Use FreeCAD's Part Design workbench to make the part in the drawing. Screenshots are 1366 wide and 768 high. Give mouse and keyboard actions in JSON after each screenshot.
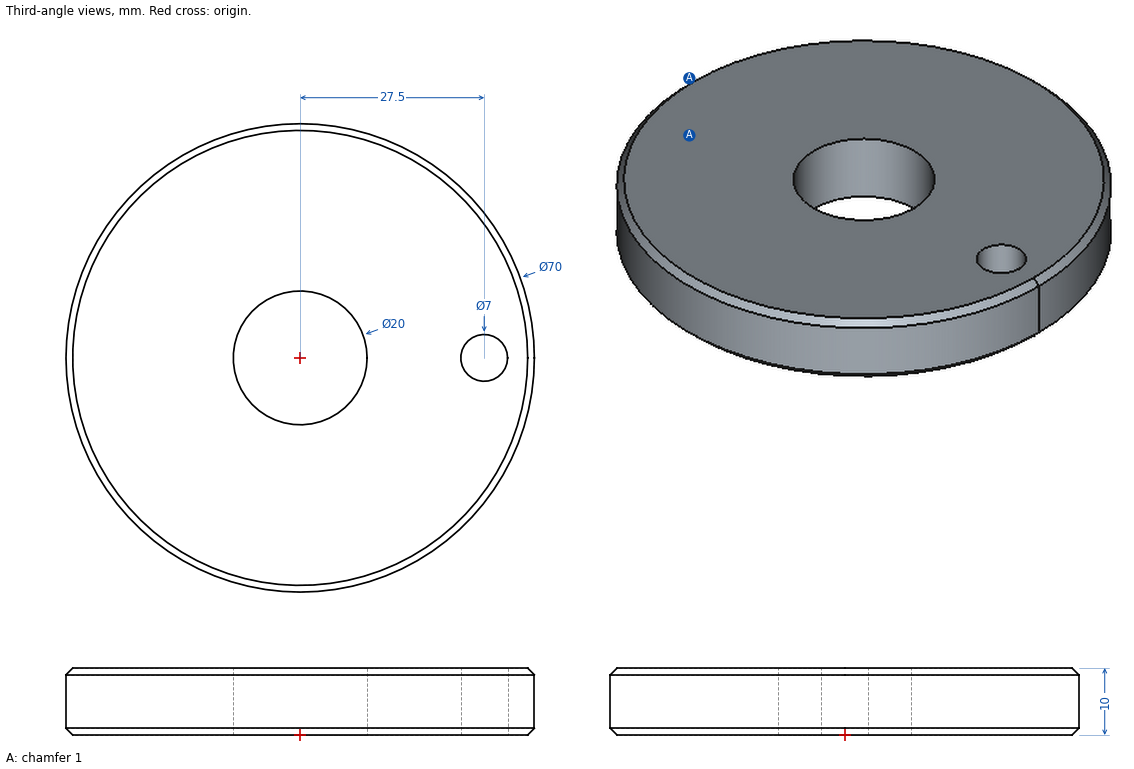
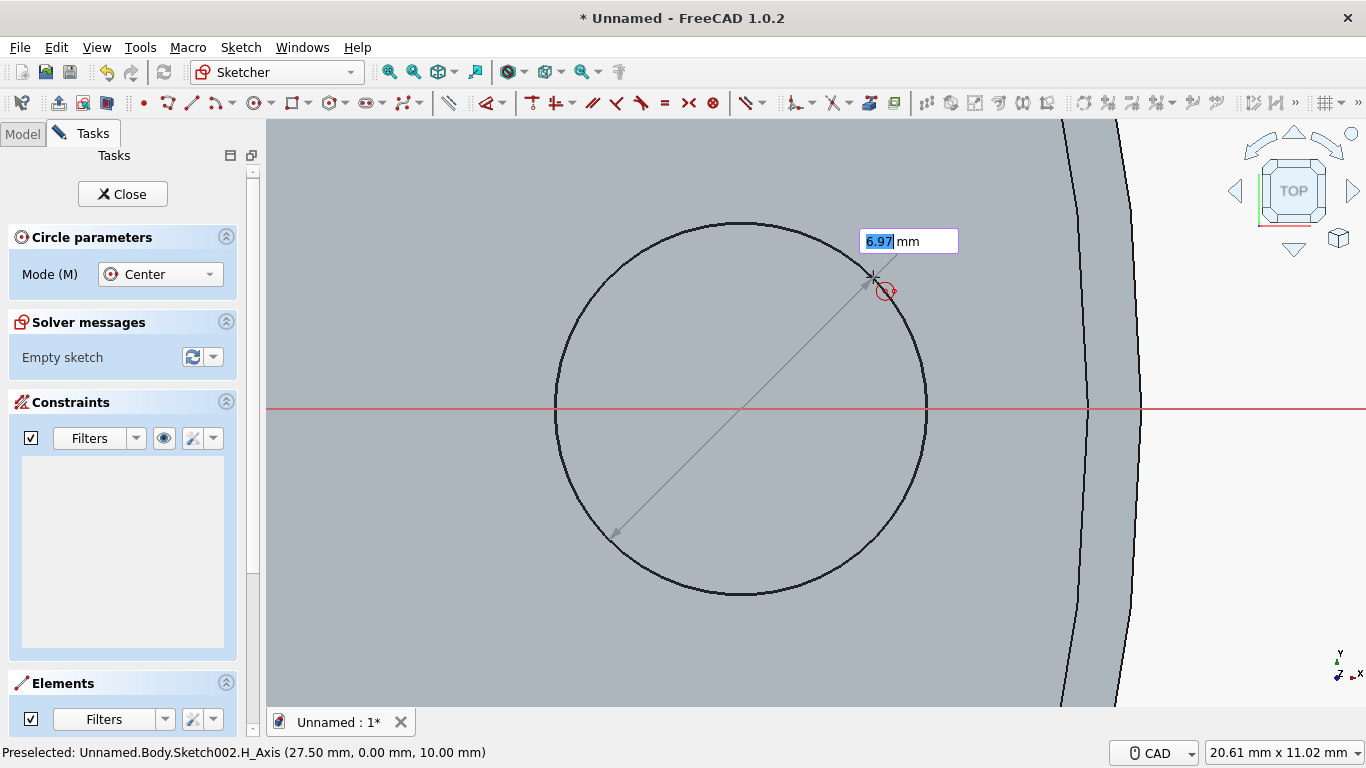
{"action": "type", "text": "7"}
{"action": "key", "text": "Return"}
{"action": "key", "text": "Escape"}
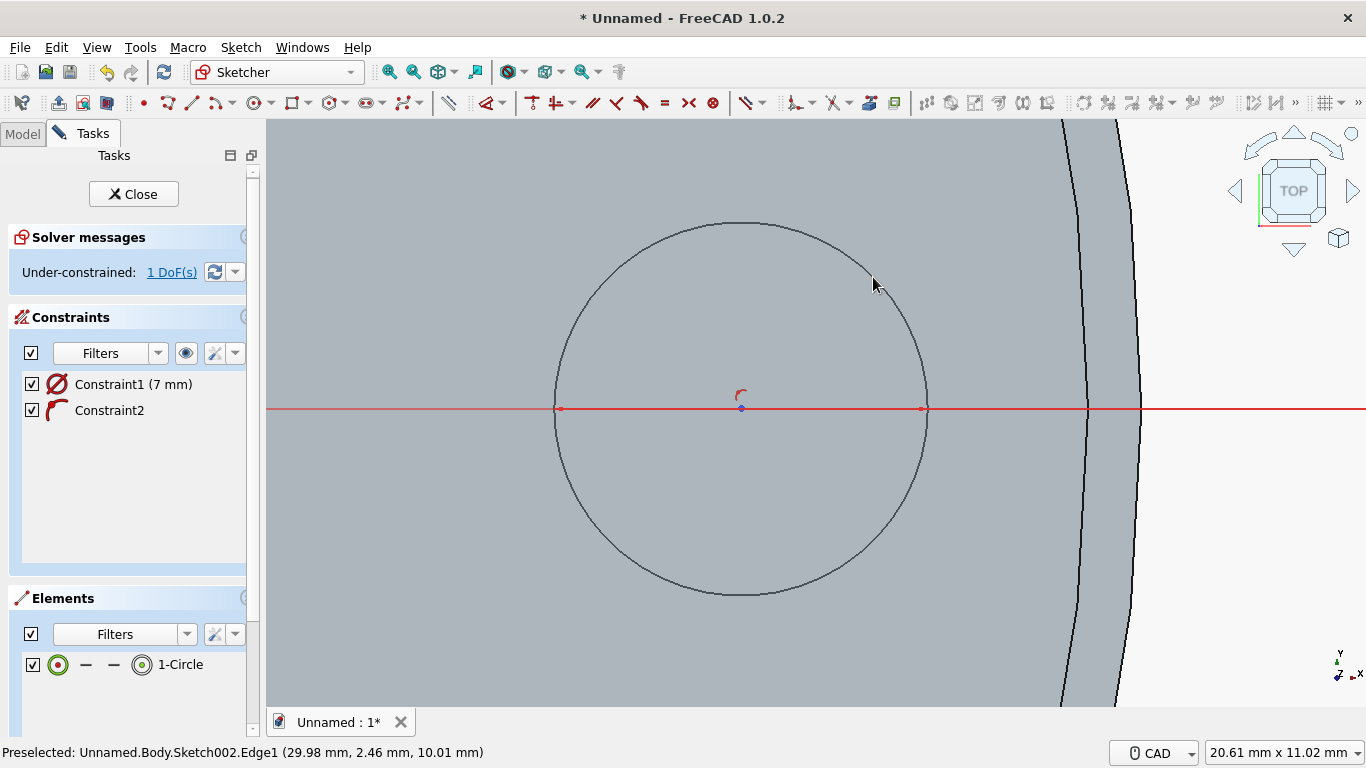
{"action": "left_click", "coordinate": [741, 409]}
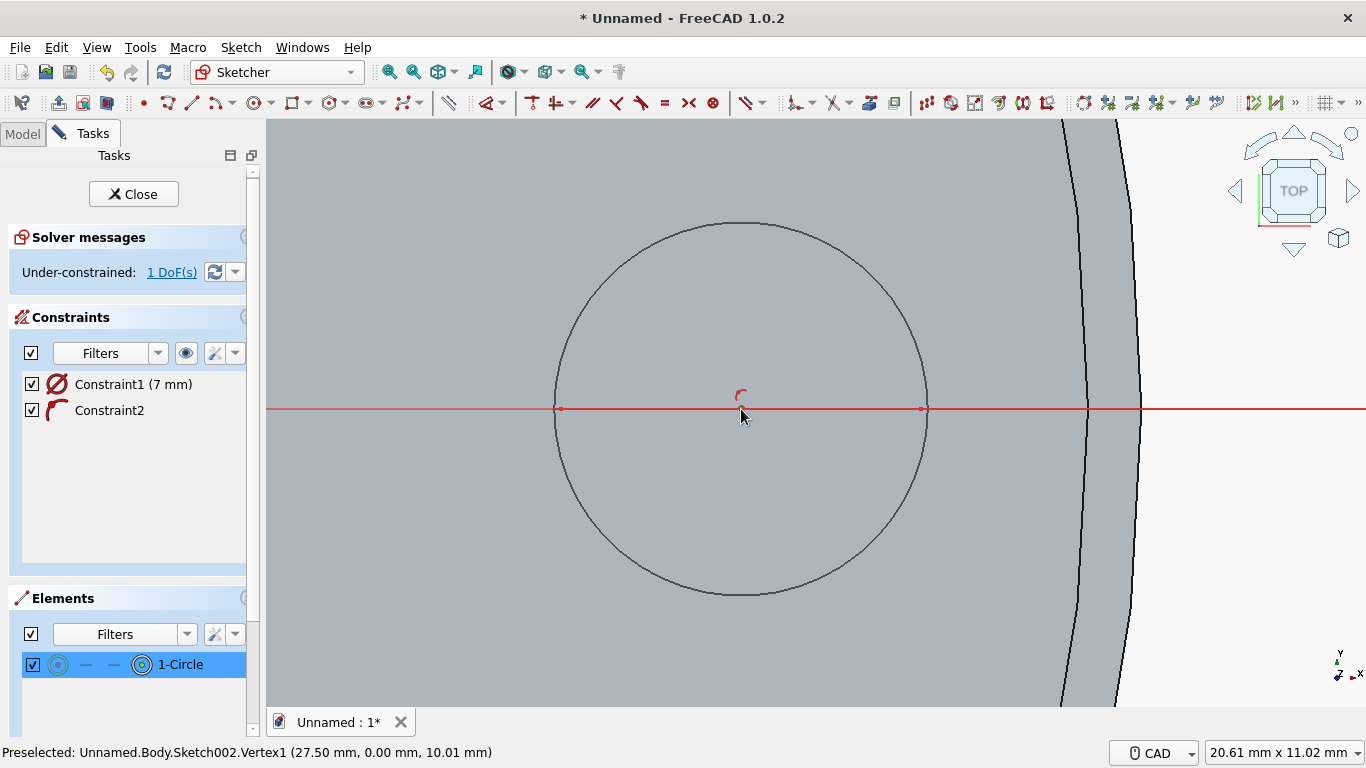
{"action": "key", "text": "l"}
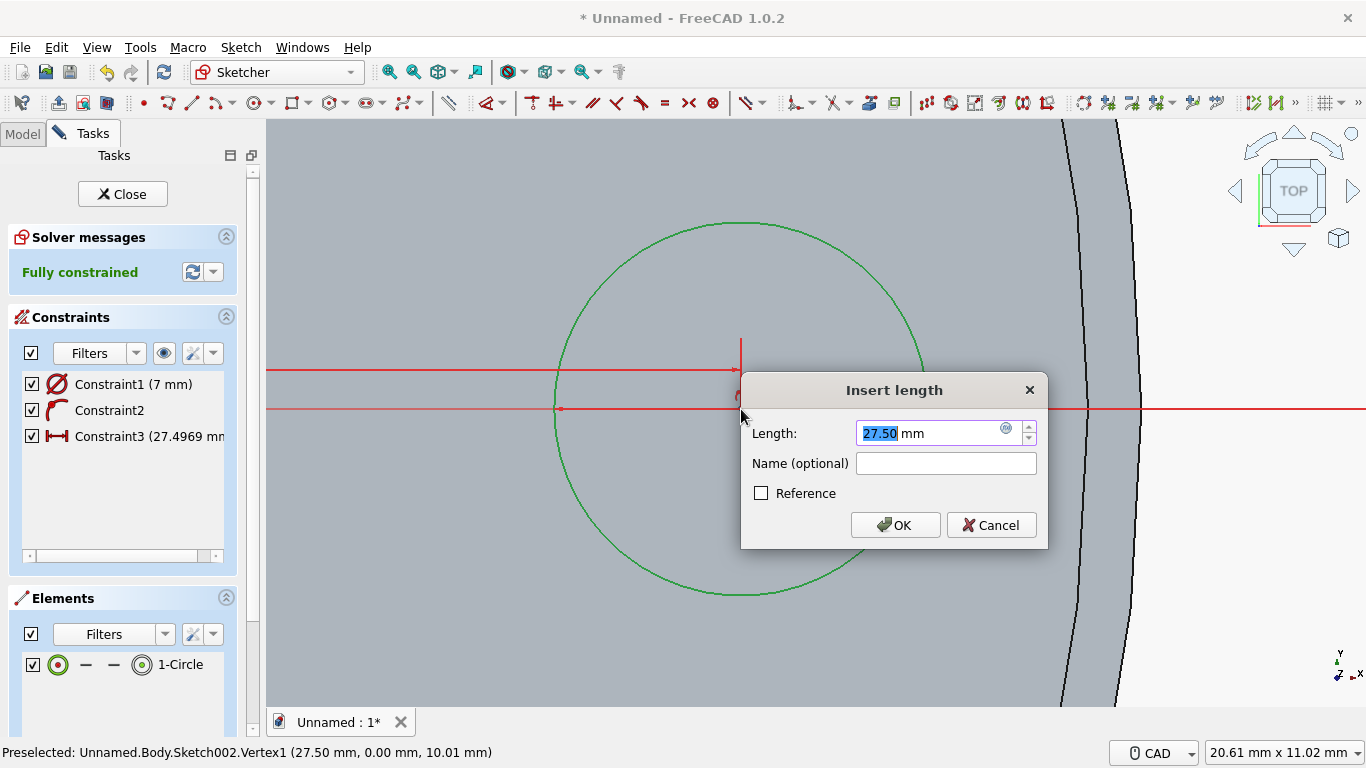
{"action": "type", "text": "27.5"}
{"action": "key", "text": "Return"}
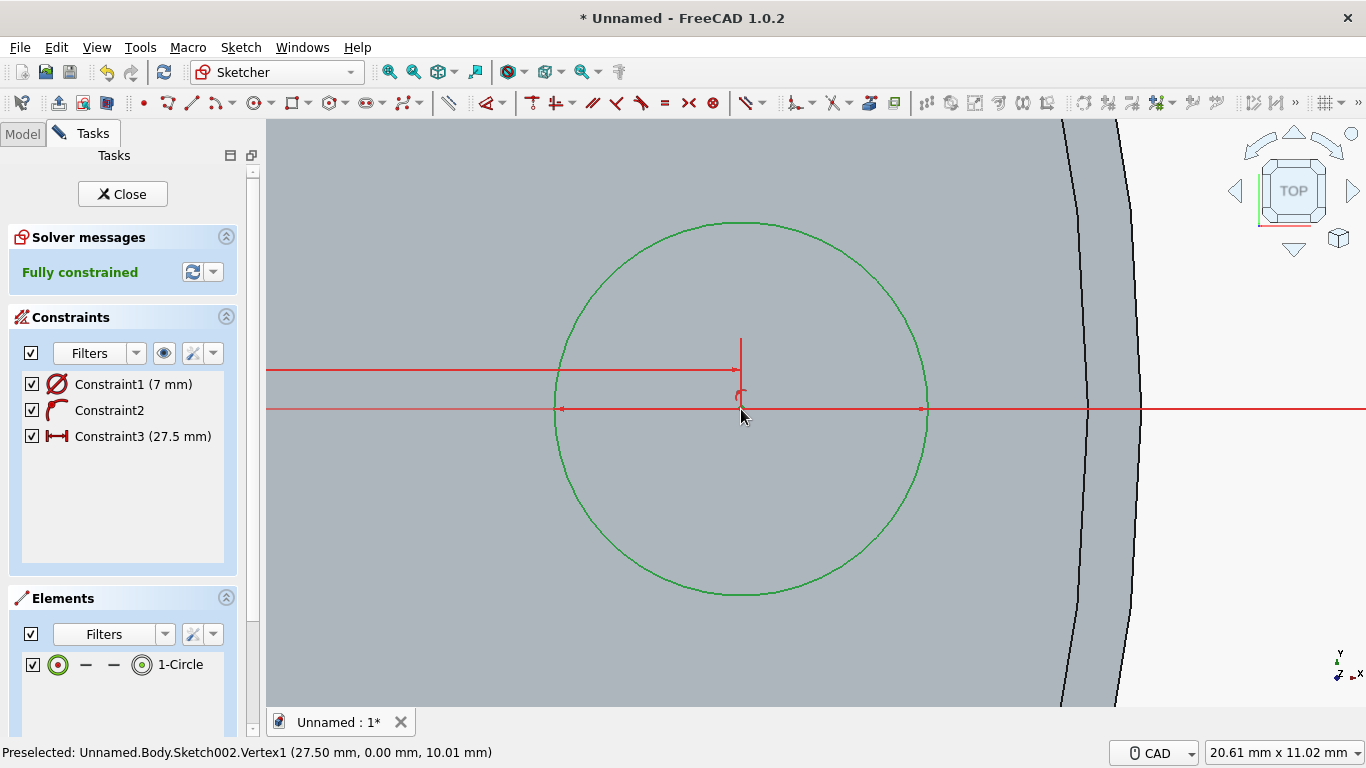
{"action": "left_click", "coordinate": [123, 194]}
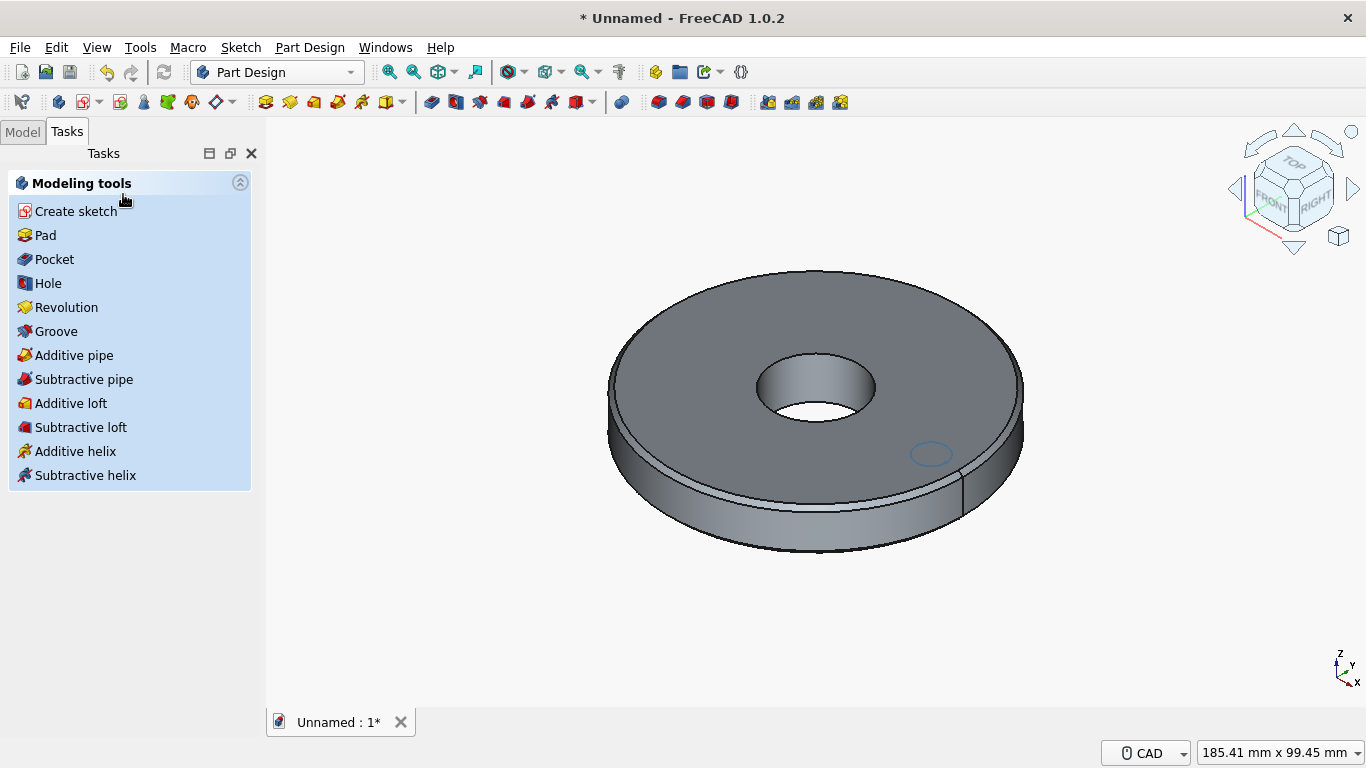
{"action": "left_click", "coordinate": [432, 102]}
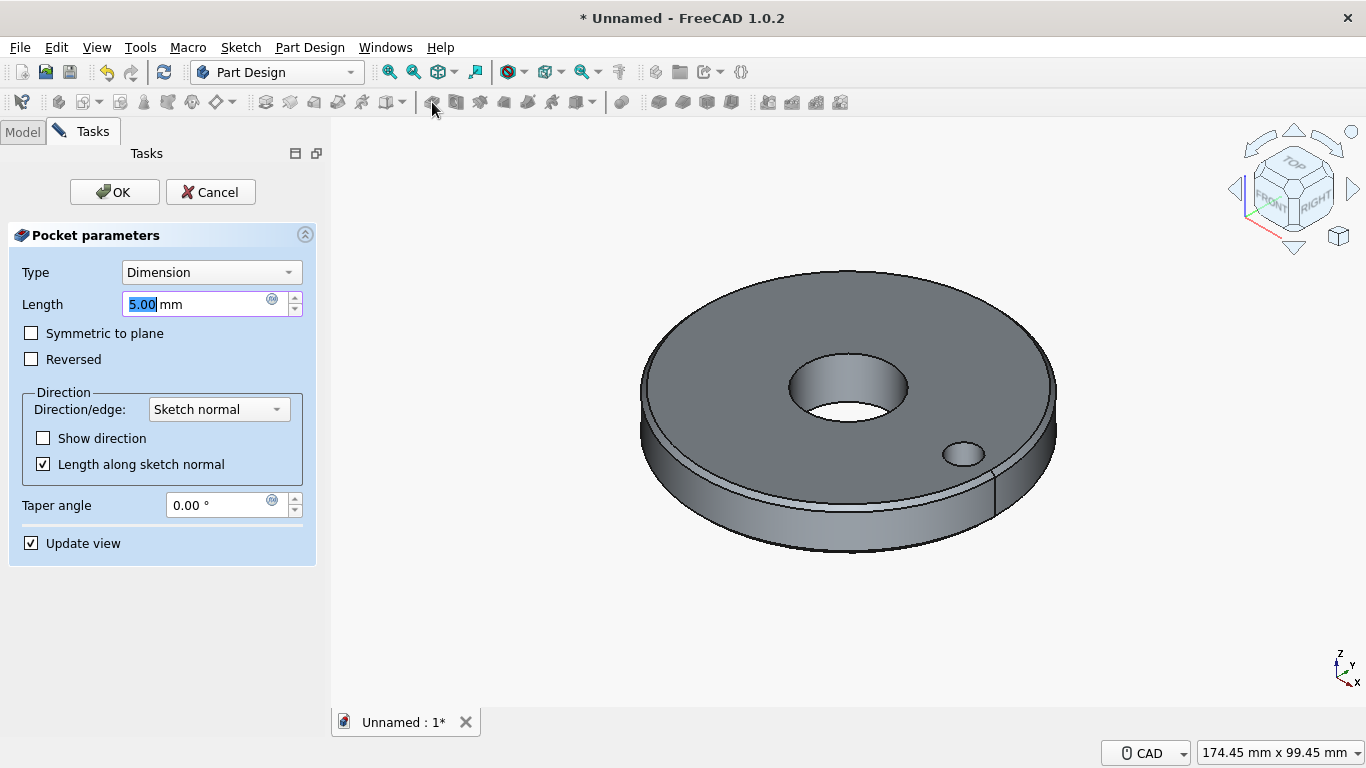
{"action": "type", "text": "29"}
{"action": "key", "text": "Tab"}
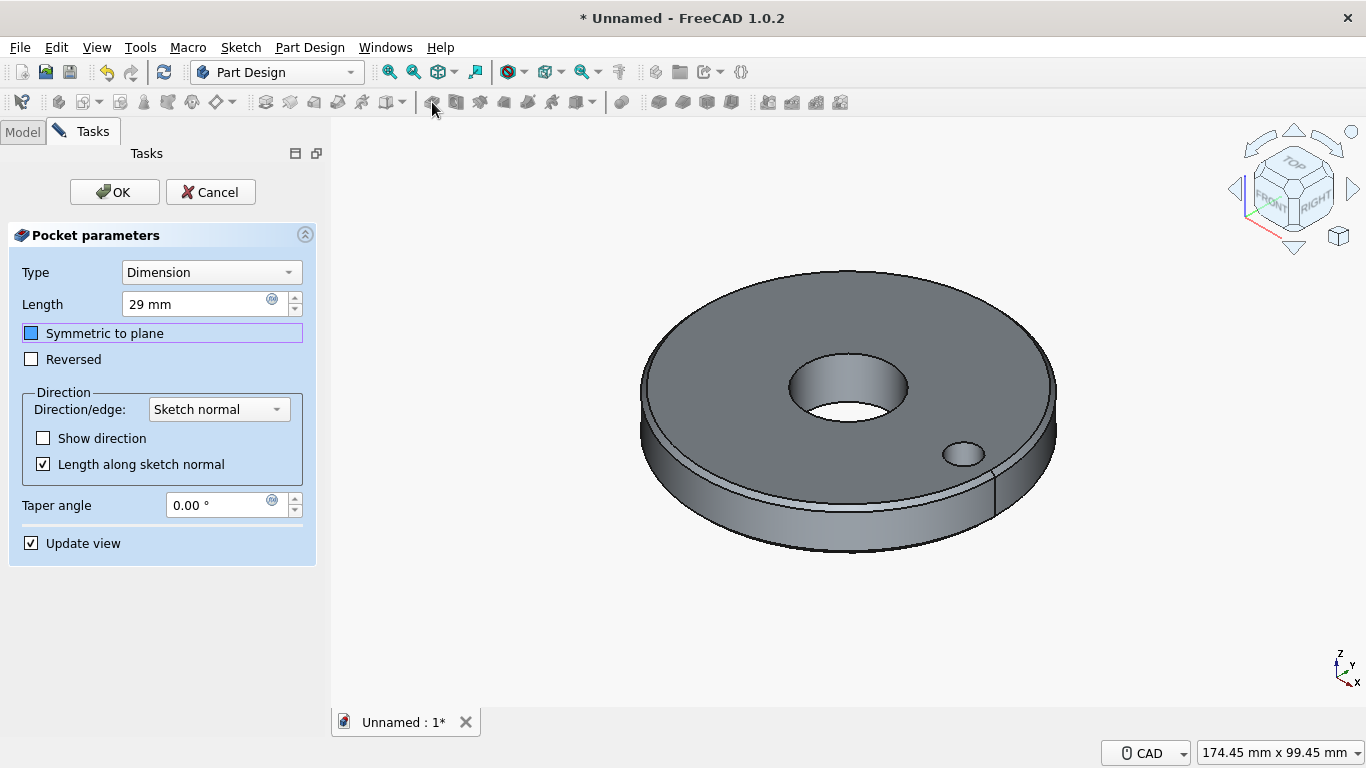
{"action": "left_click", "coordinate": [115, 192]}